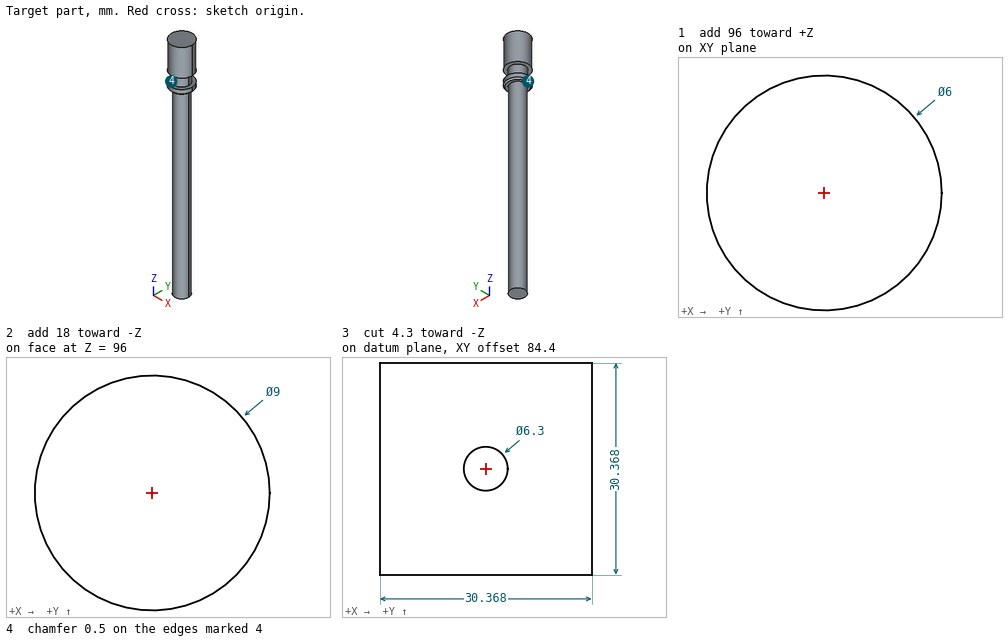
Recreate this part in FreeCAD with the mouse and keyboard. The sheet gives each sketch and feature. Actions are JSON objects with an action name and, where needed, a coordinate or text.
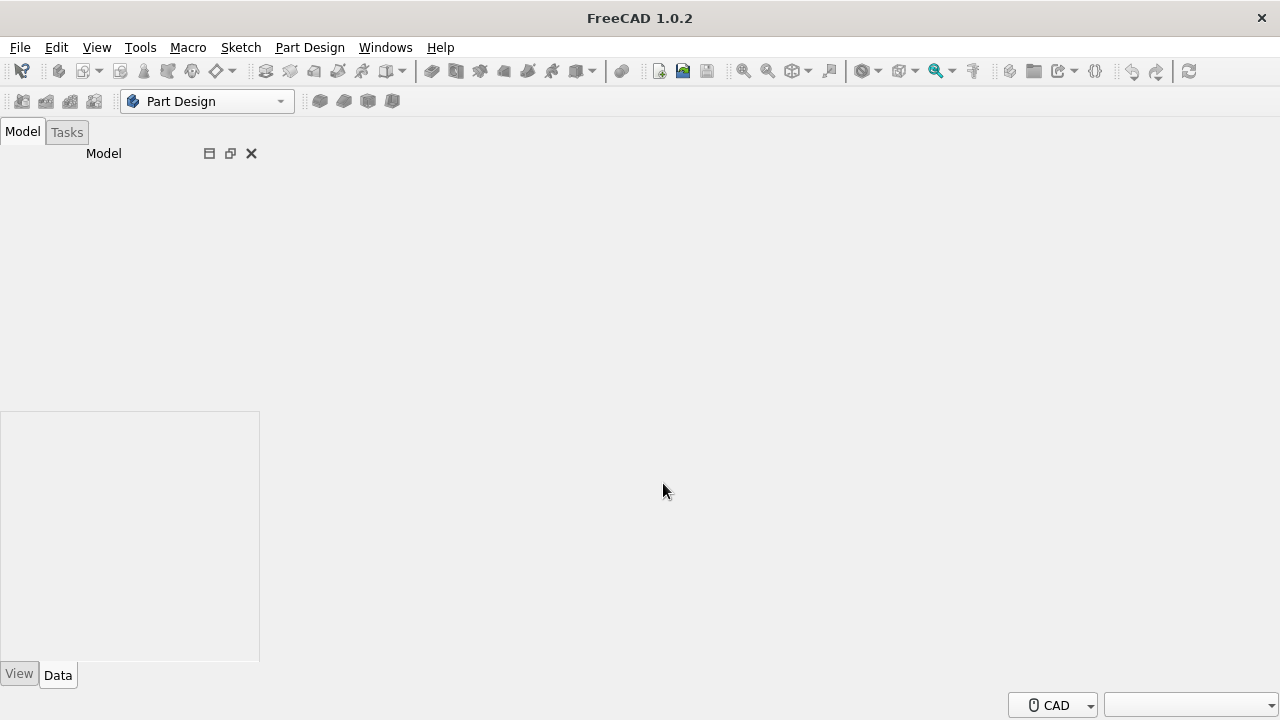
{"action": "key", "text": "ctrl+n"}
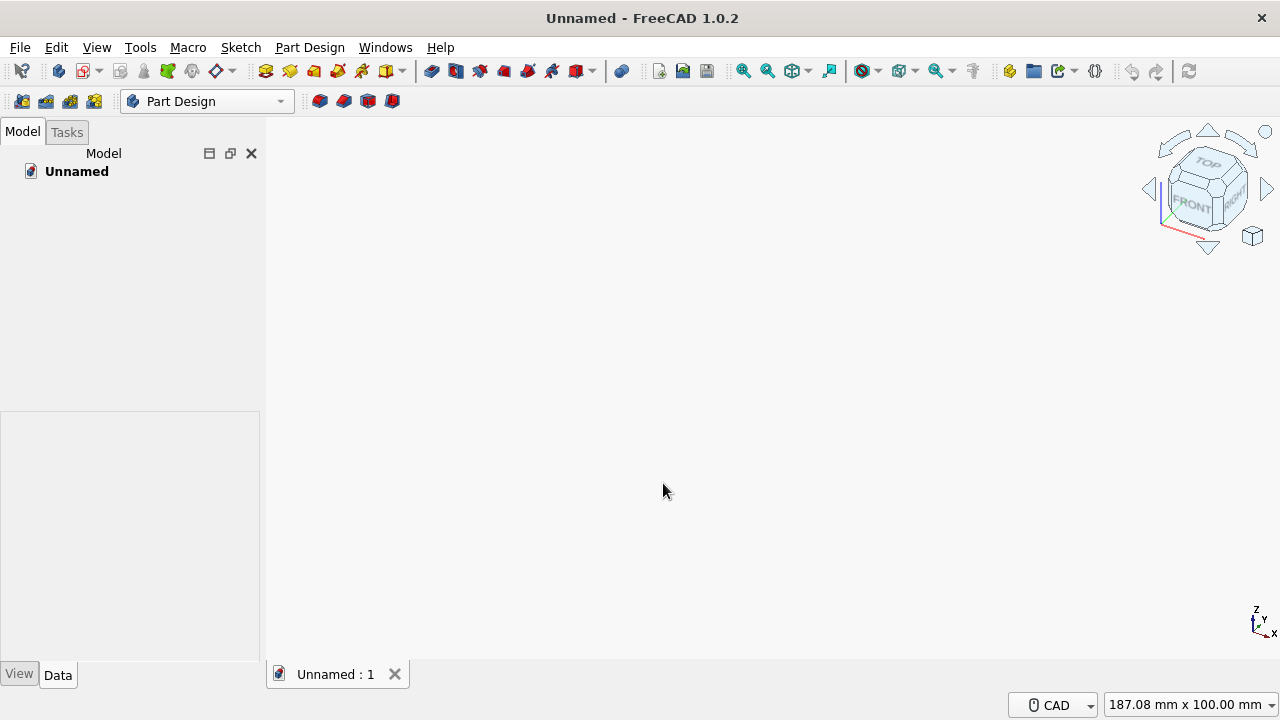
{"action": "left_click", "coordinate": [84, 72]}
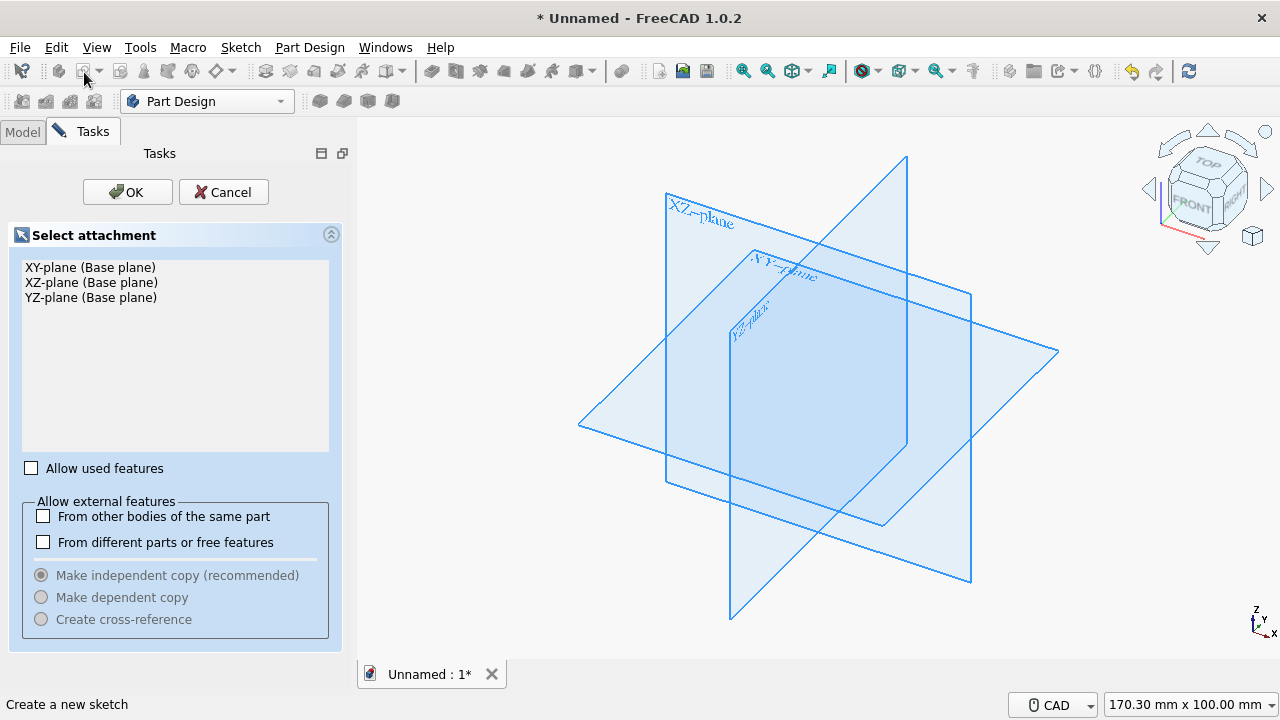
{"action": "left_click", "coordinate": [82, 268]}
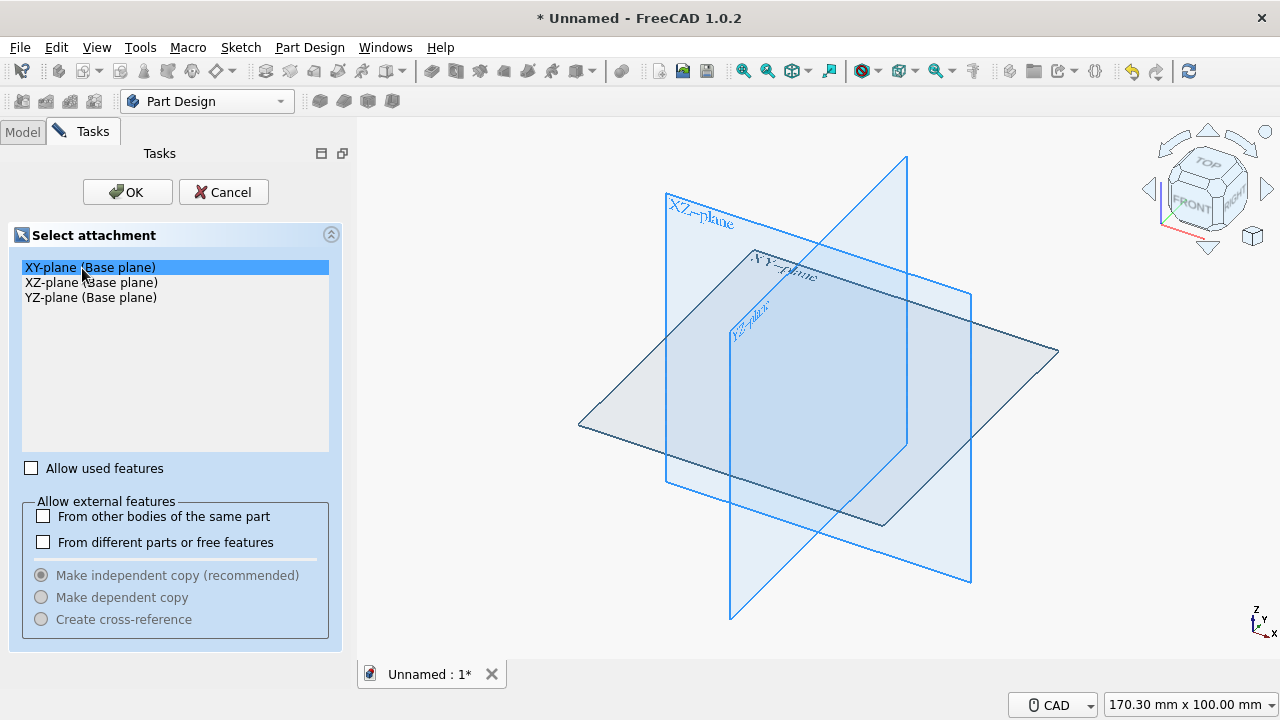
{"action": "left_click", "coordinate": [128, 192]}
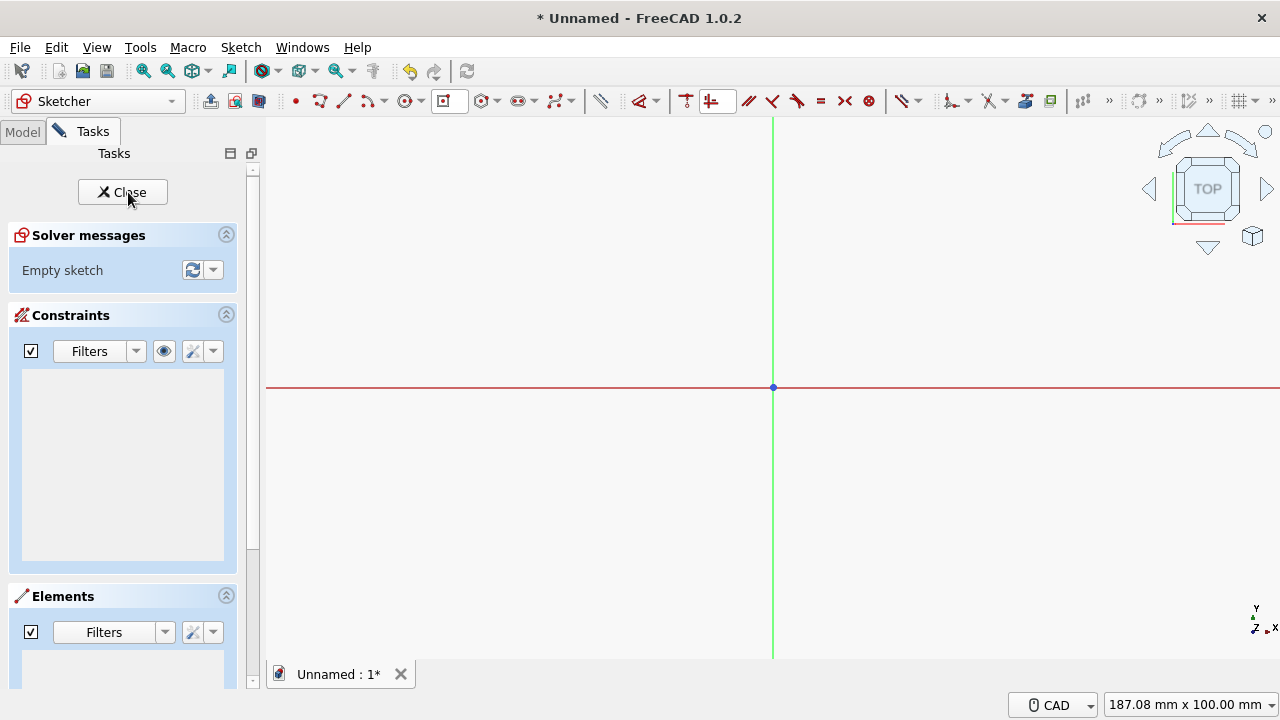
{"action": "scroll", "coordinate": [780, 388], "scroll_direction": "up", "scroll_amount": 12}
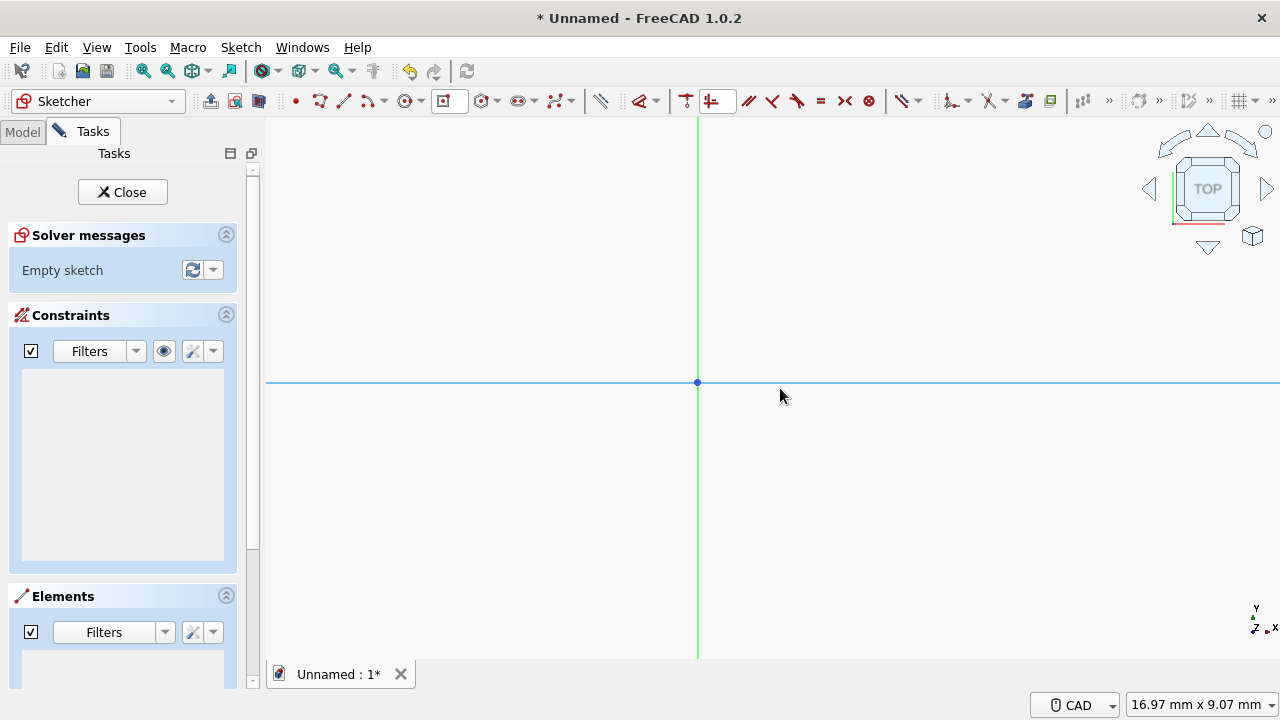
{"action": "key", "text": "g c"}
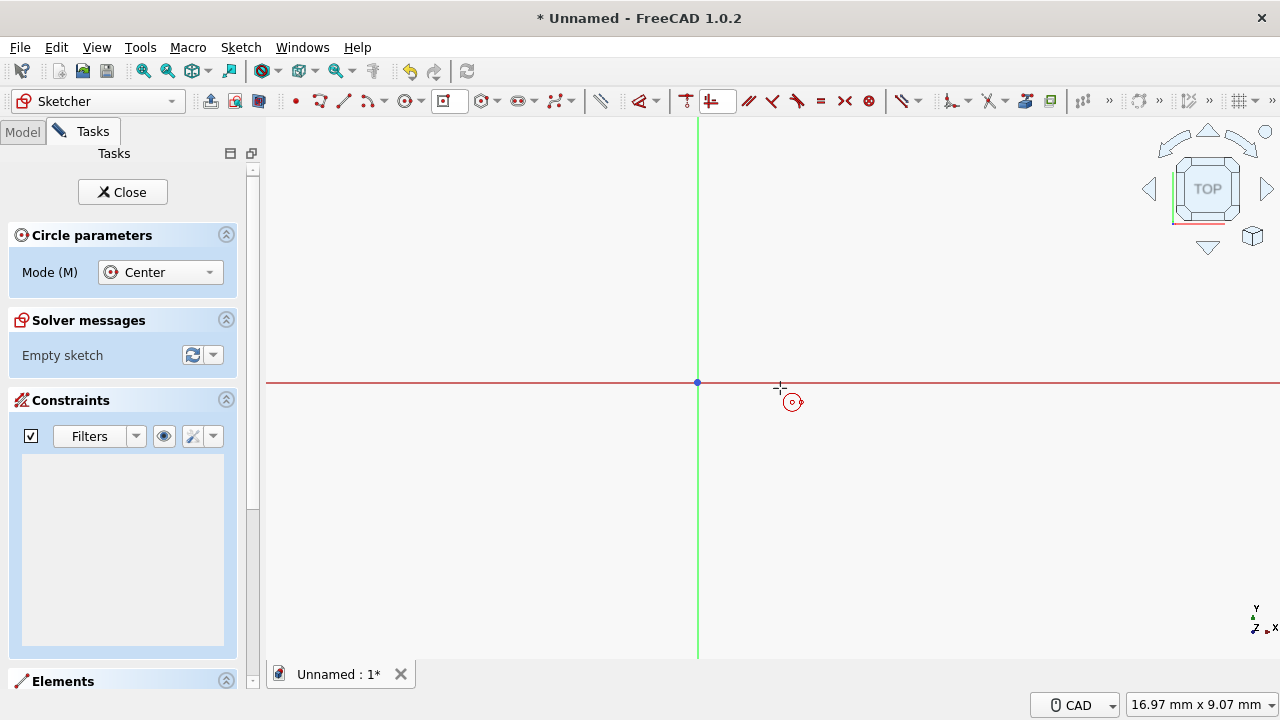
{"action": "left_click", "coordinate": [698, 383]}
{"action": "left_click", "coordinate": [824, 256]}
{"action": "key", "text": "Escape"}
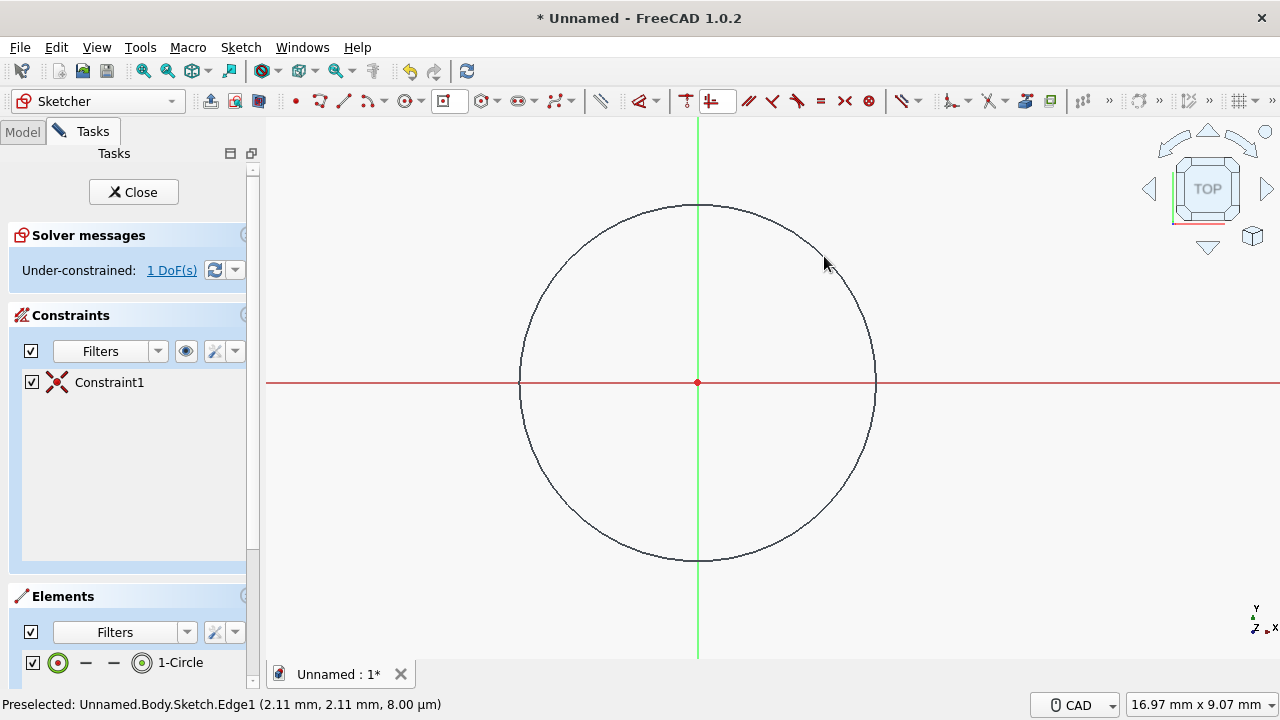
{"action": "left_click", "coordinate": [640, 102]}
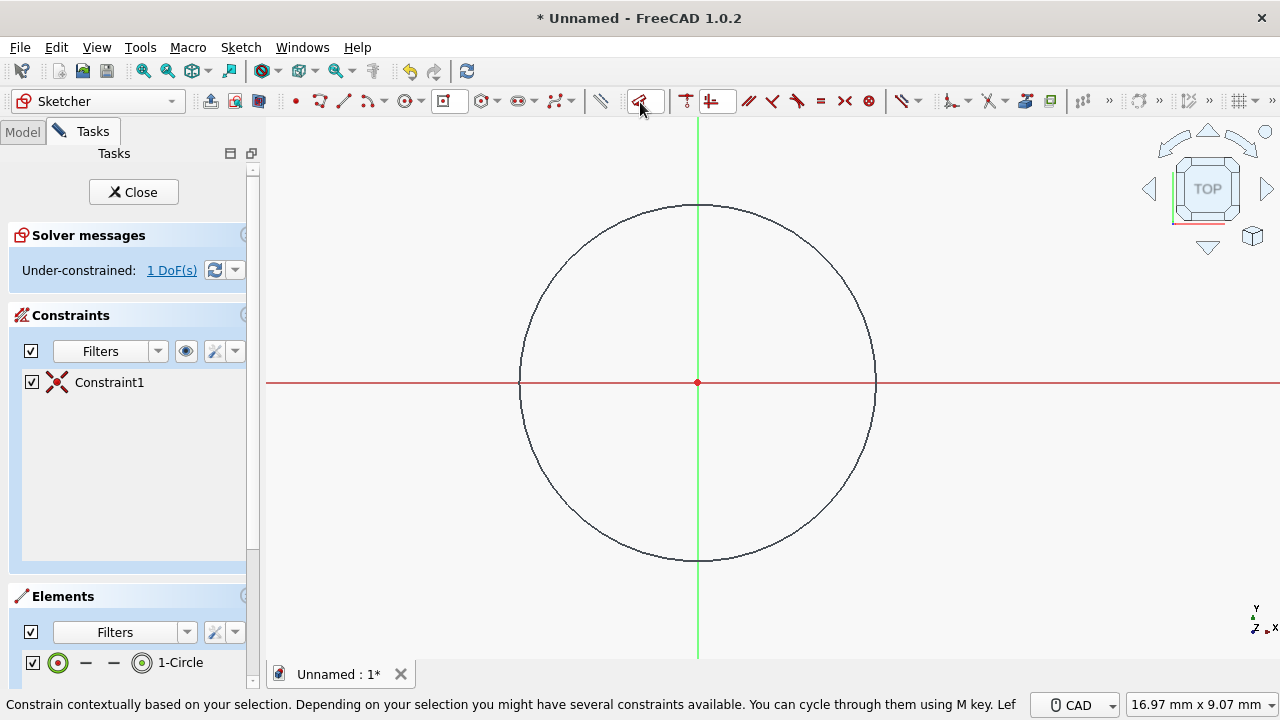
{"action": "left_click", "coordinate": [823, 256]}
{"action": "left_click", "coordinate": [845, 233]}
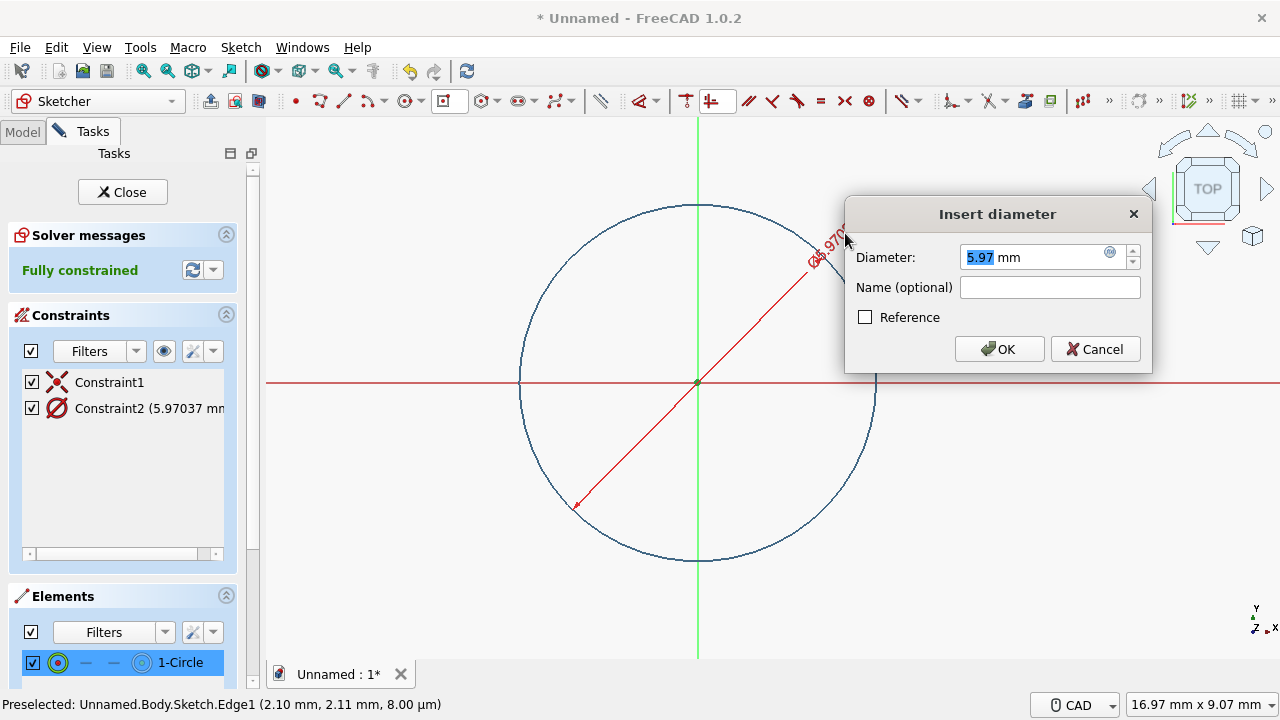
{"action": "type", "text": "6"}
{"action": "key", "text": "Return"}
{"action": "key", "text": "Escape"}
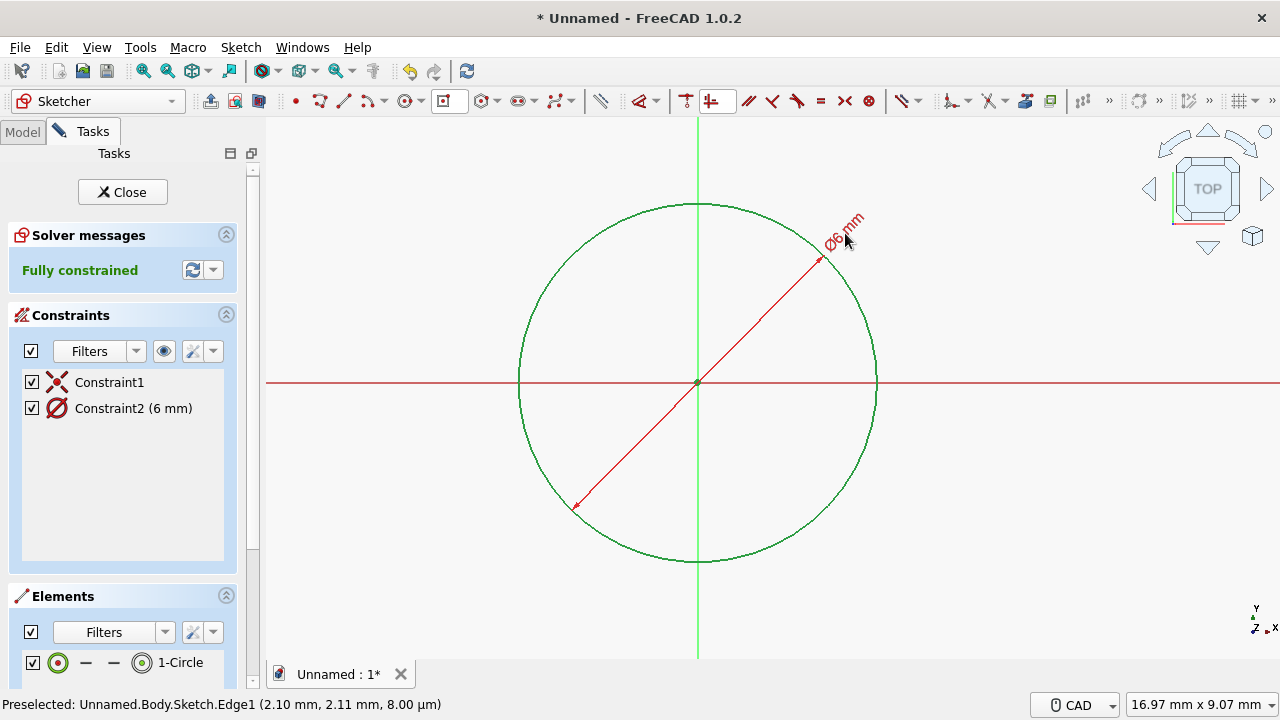
{"action": "left_click", "coordinate": [123, 192]}